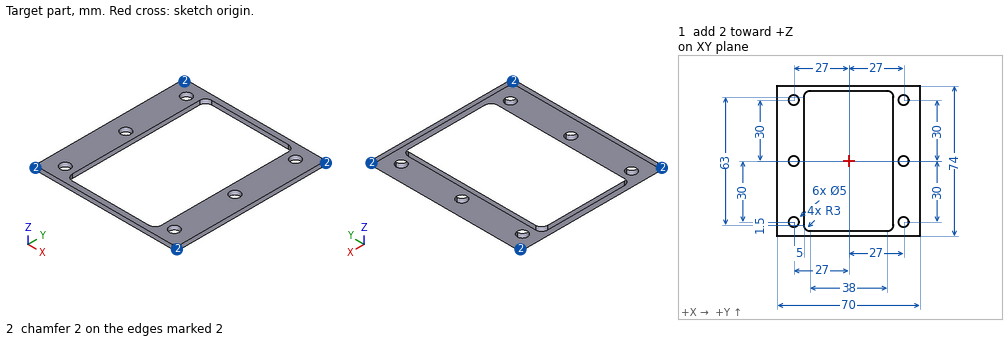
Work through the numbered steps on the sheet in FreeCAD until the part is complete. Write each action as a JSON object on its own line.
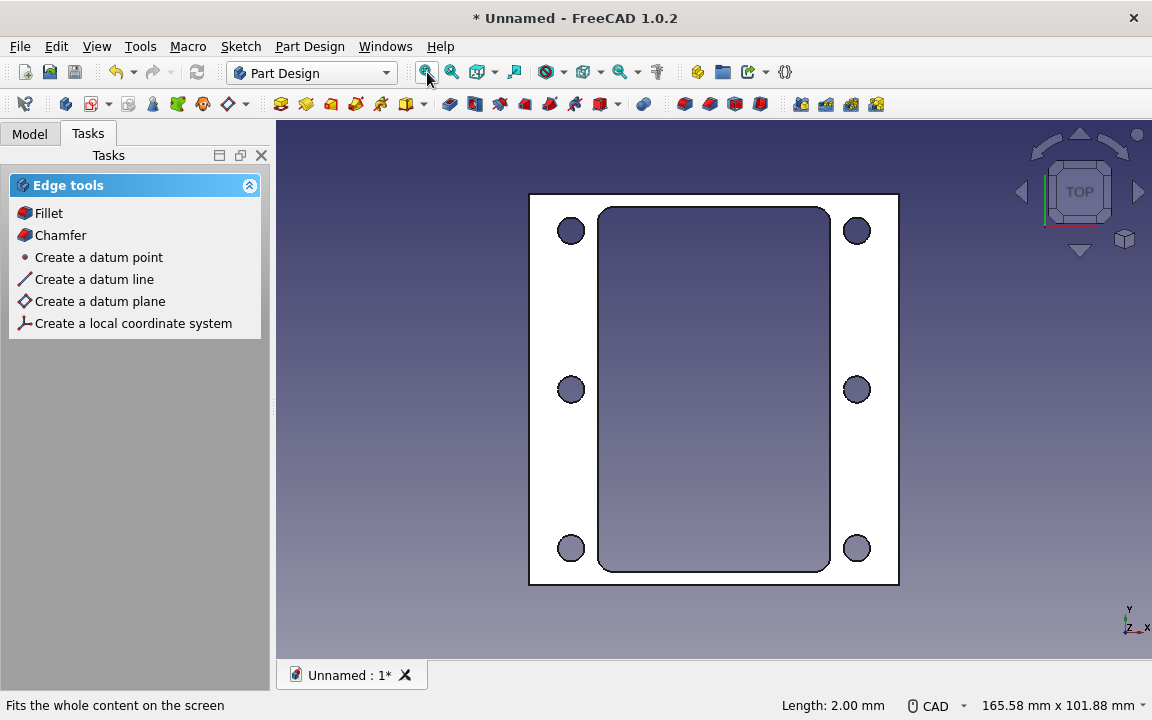
{"action": "scroll", "coordinate": [529, 584], "scroll_direction": "up", "scroll_amount": 7}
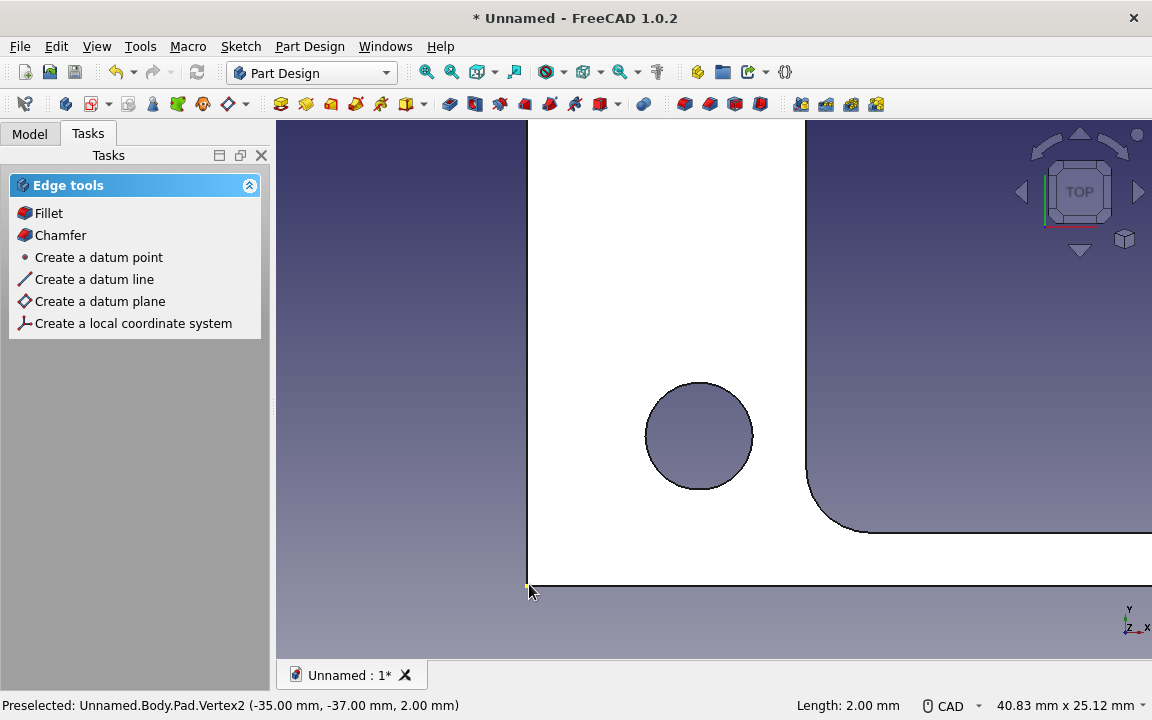
{"action": "left_click", "coordinate": [427, 72]}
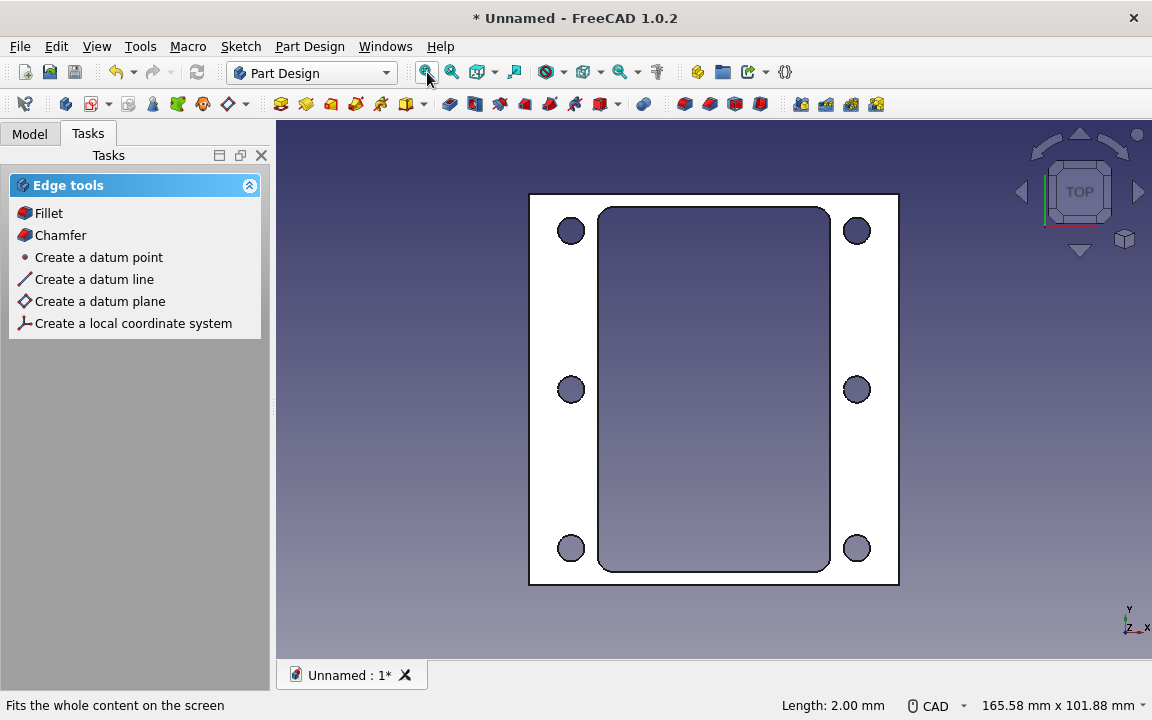
{"action": "key", "text": "1"}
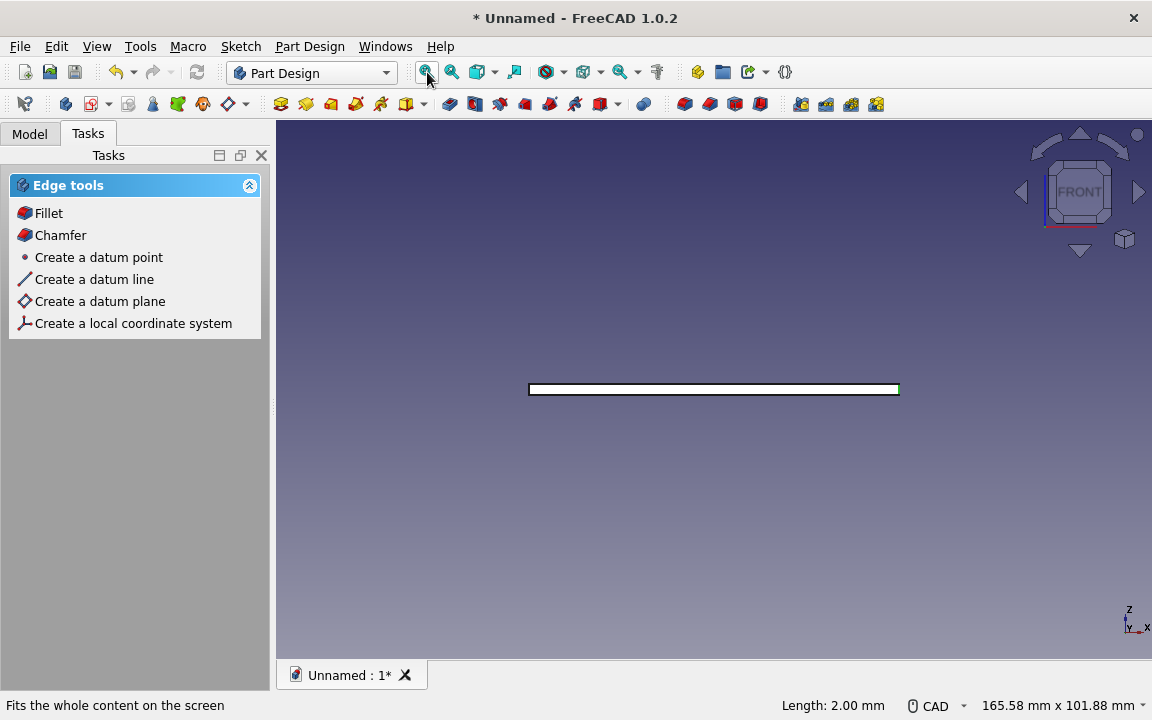
{"action": "left_click", "coordinate": [427, 72]}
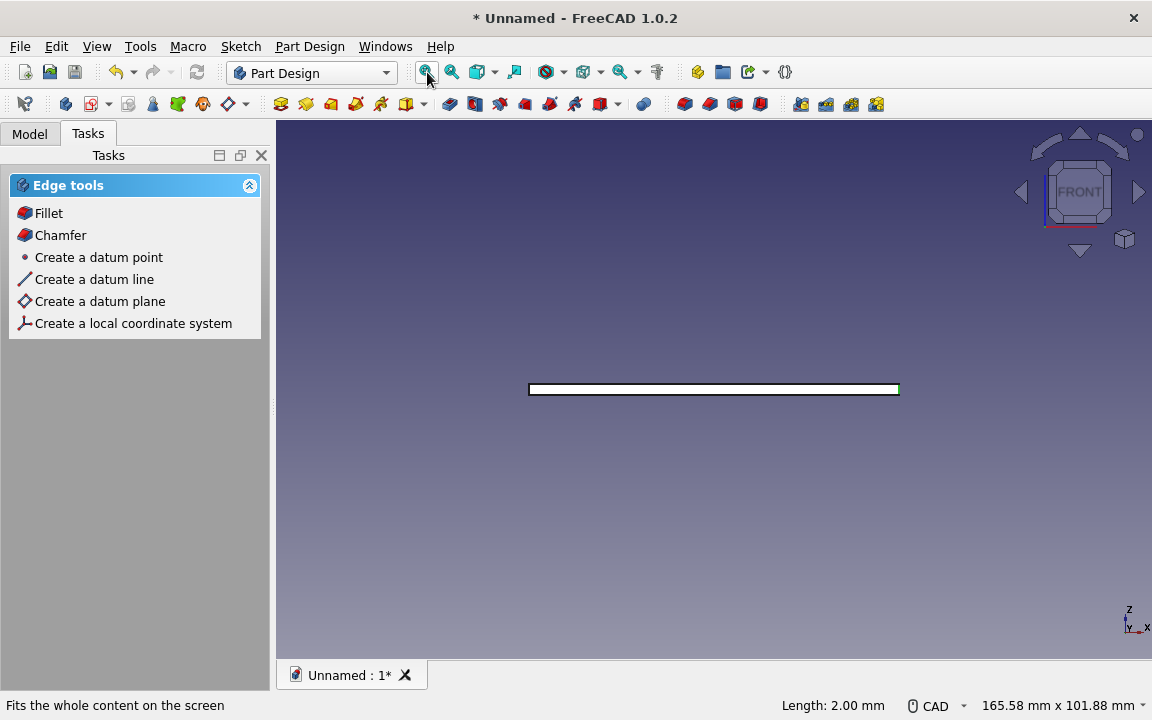
{"action": "scroll", "coordinate": [529, 389], "scroll_direction": "up", "scroll_amount": 7}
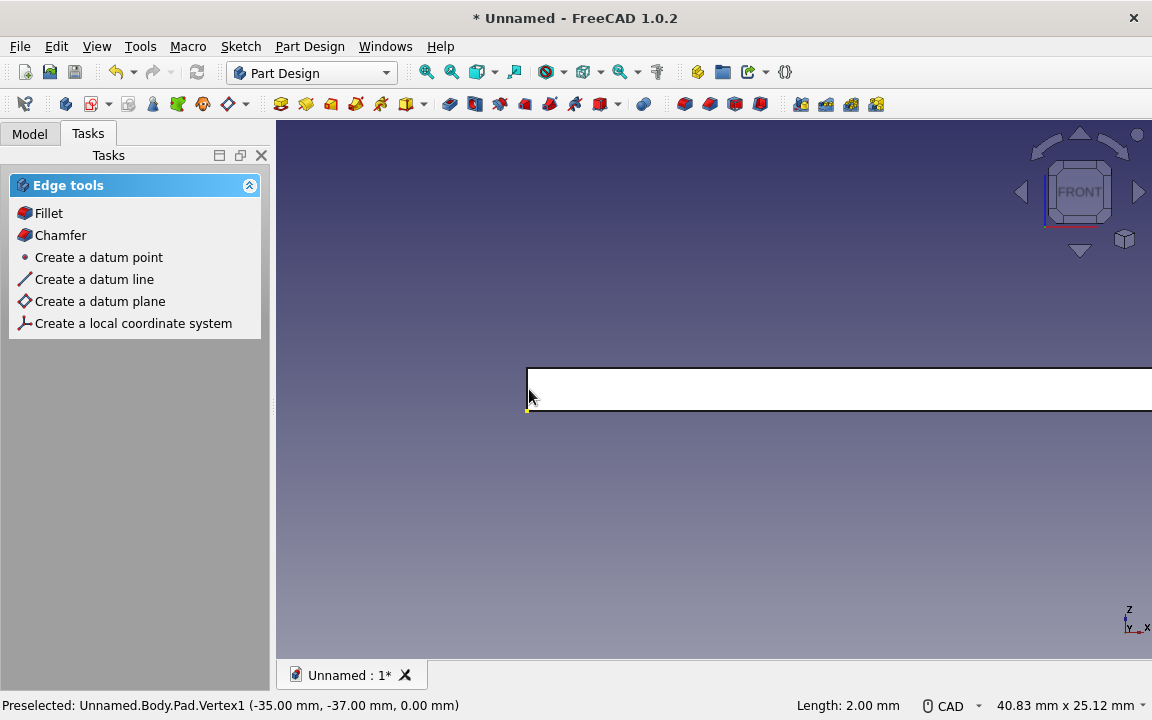
{"action": "left_click", "coordinate": [527, 389], "text": "ctrl"}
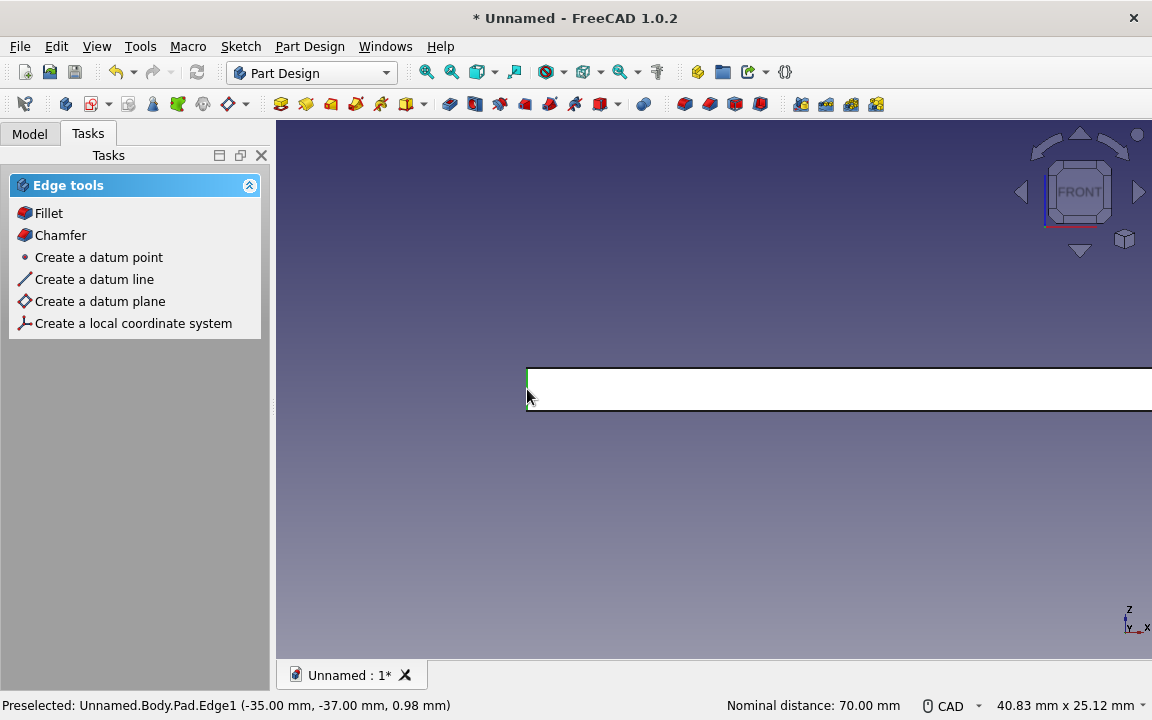
{"action": "left_click", "coordinate": [427, 72]}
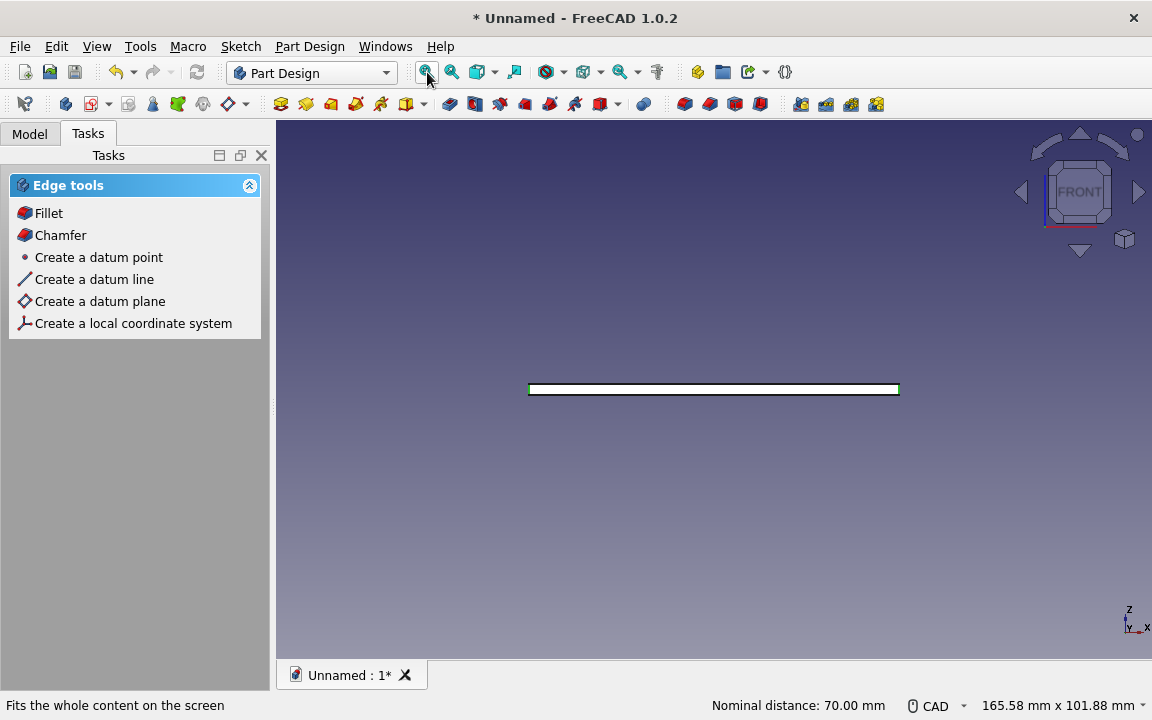
{"action": "key", "text": "3"}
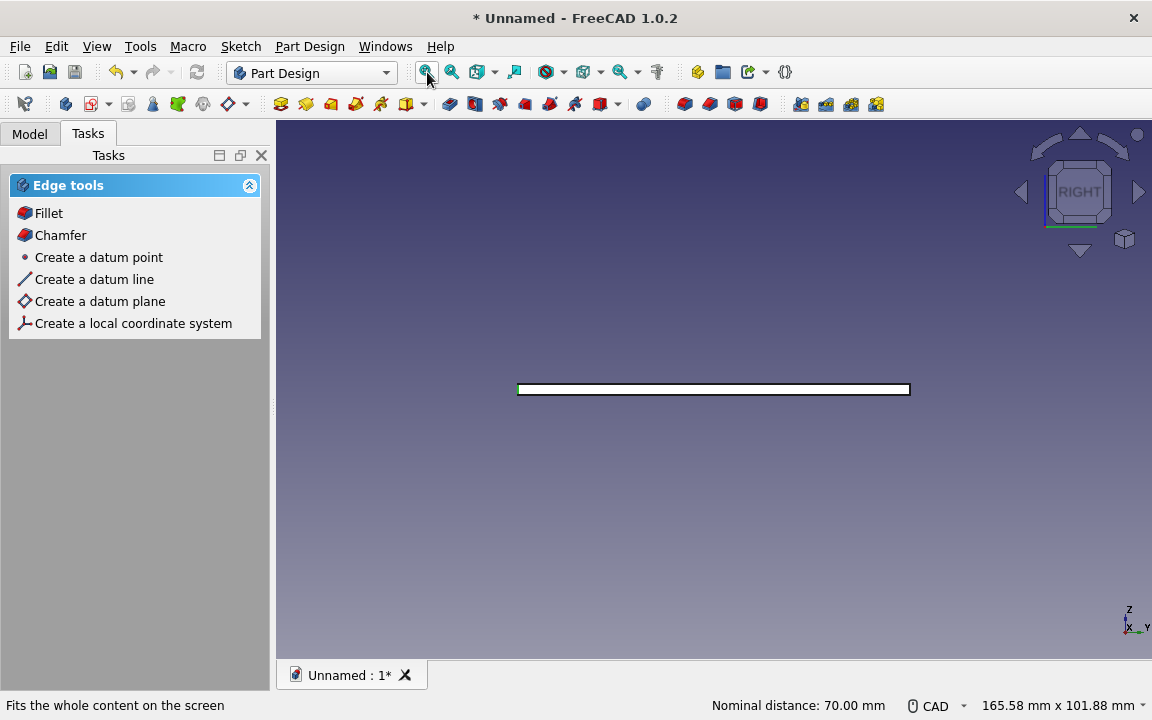
{"action": "left_click", "coordinate": [427, 72]}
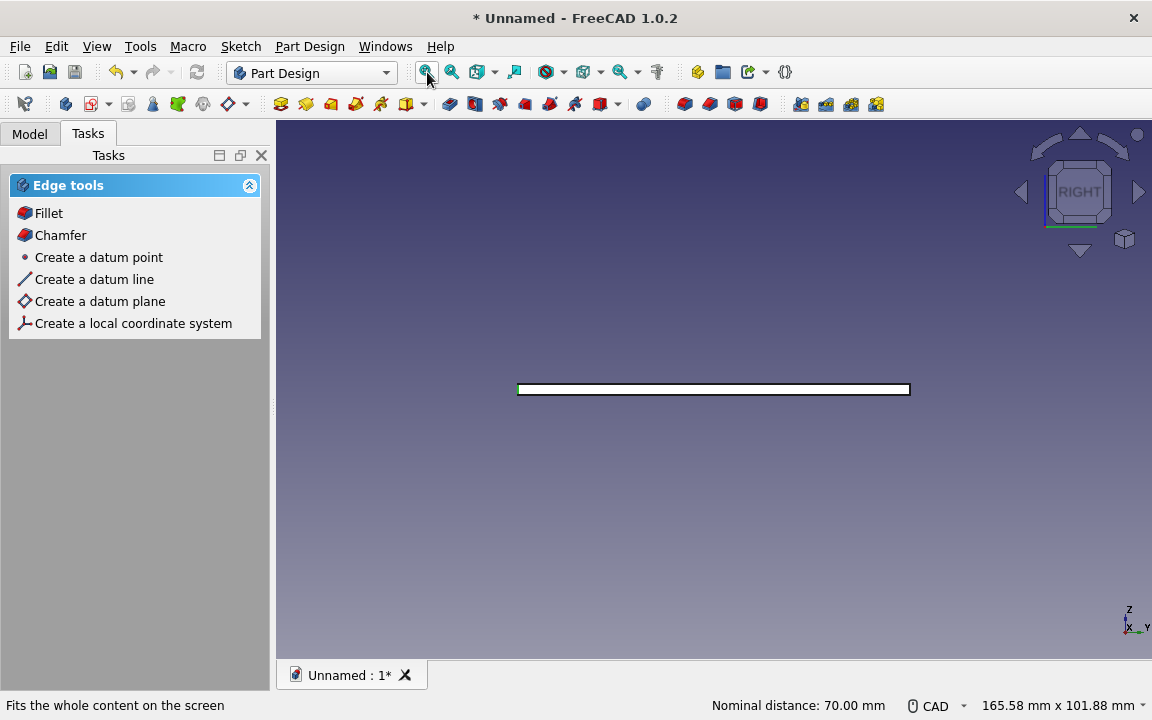
{"action": "scroll", "coordinate": [910, 388], "scroll_direction": "up", "scroll_amount": 7}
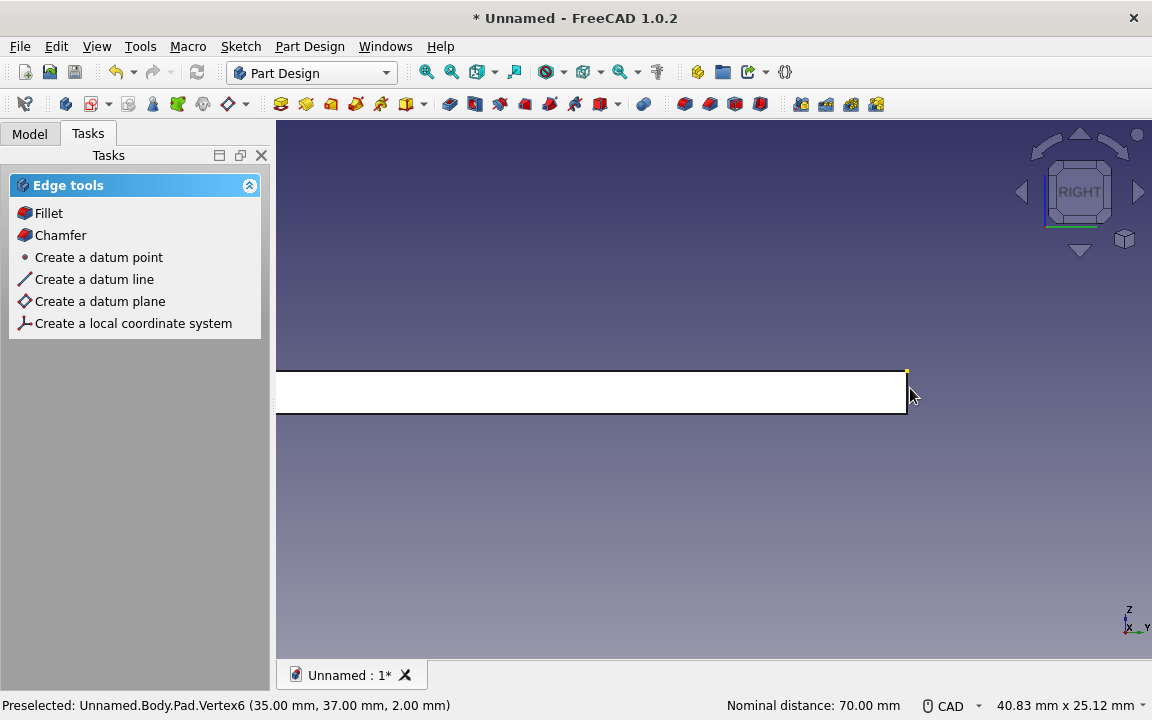
{"action": "left_click", "coordinate": [907, 392], "text": "ctrl"}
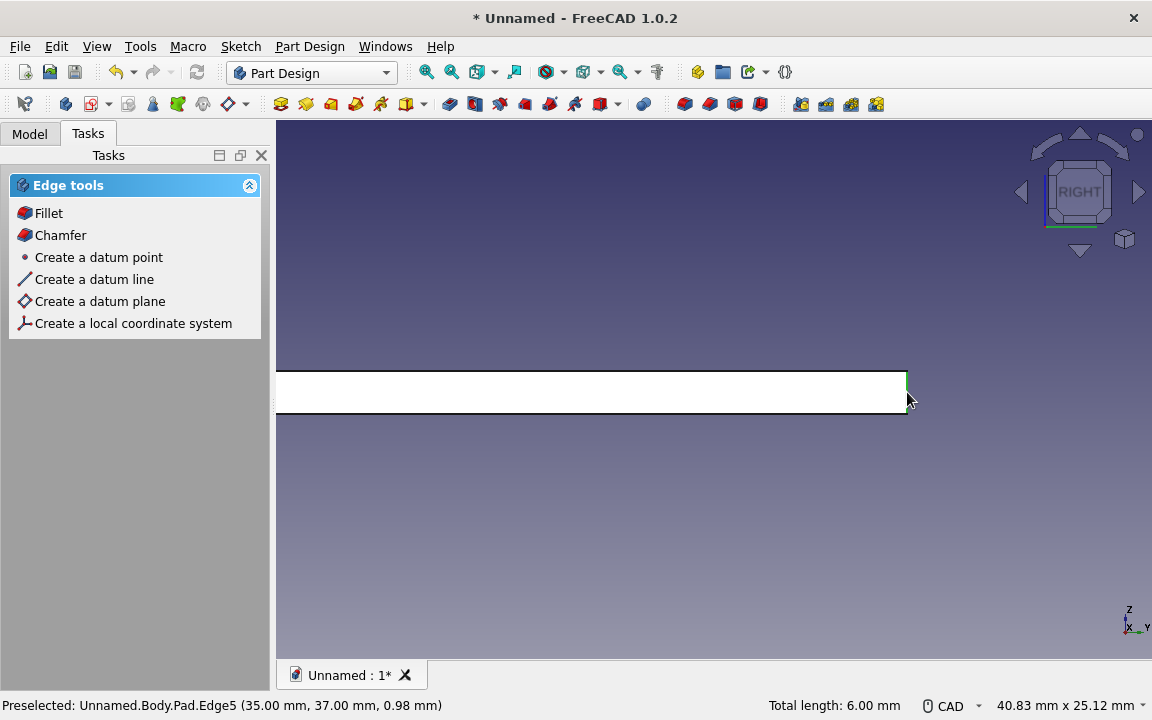
{"action": "left_click", "coordinate": [427, 72]}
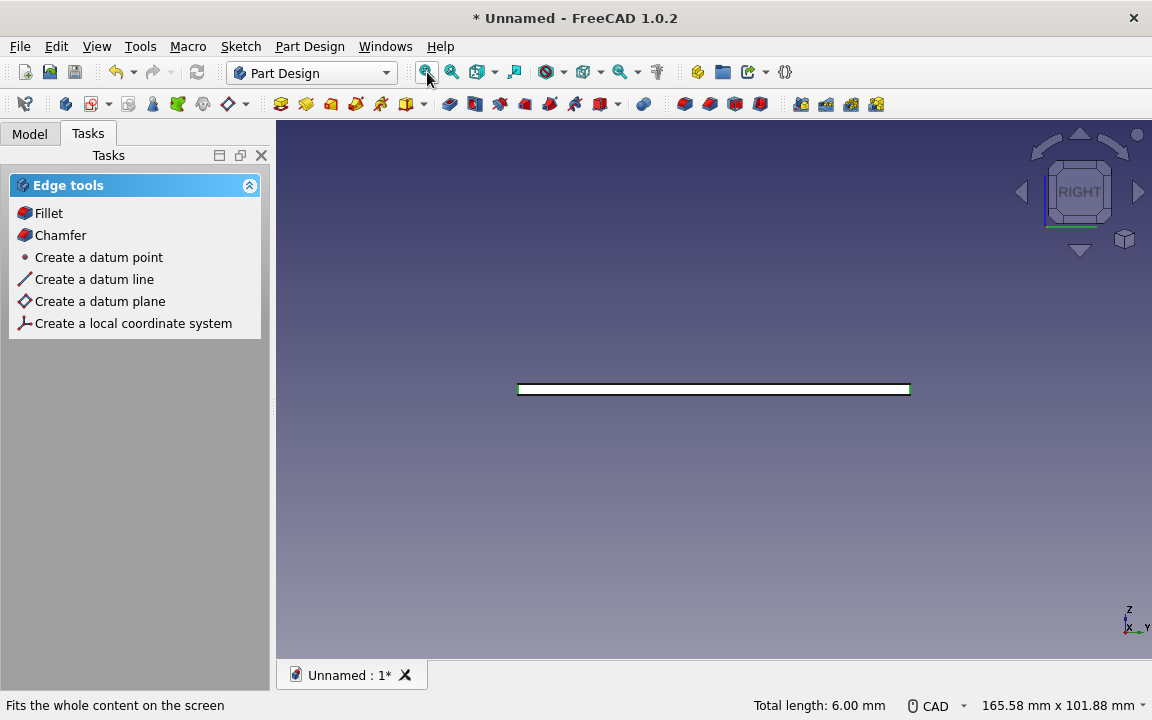
{"action": "key", "text": "5"}